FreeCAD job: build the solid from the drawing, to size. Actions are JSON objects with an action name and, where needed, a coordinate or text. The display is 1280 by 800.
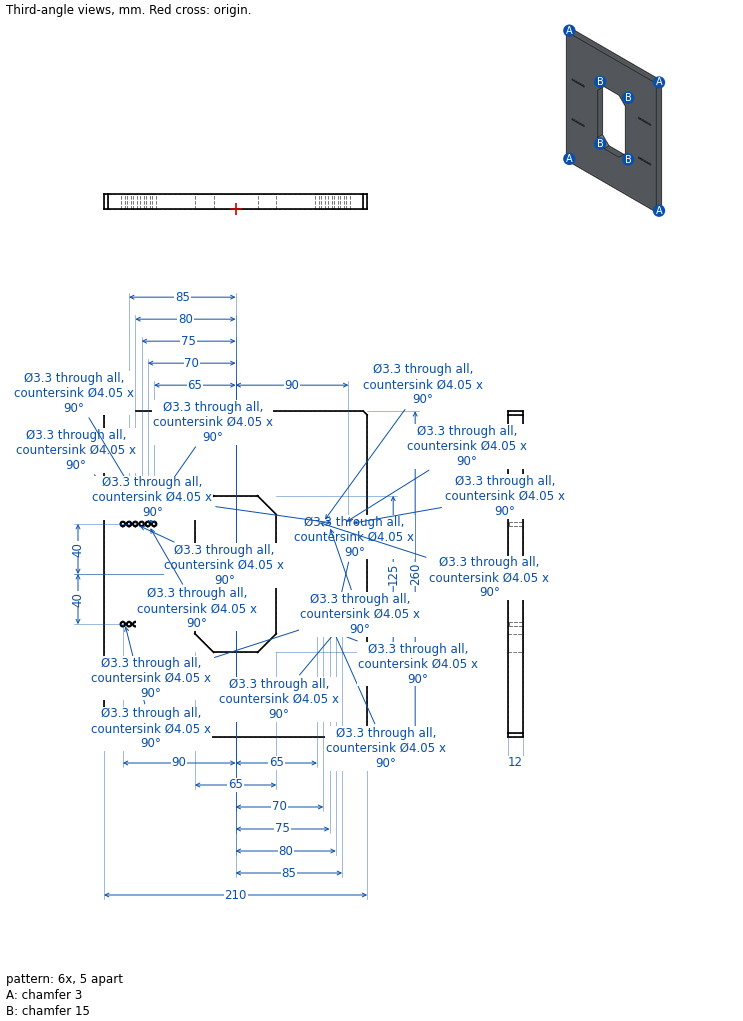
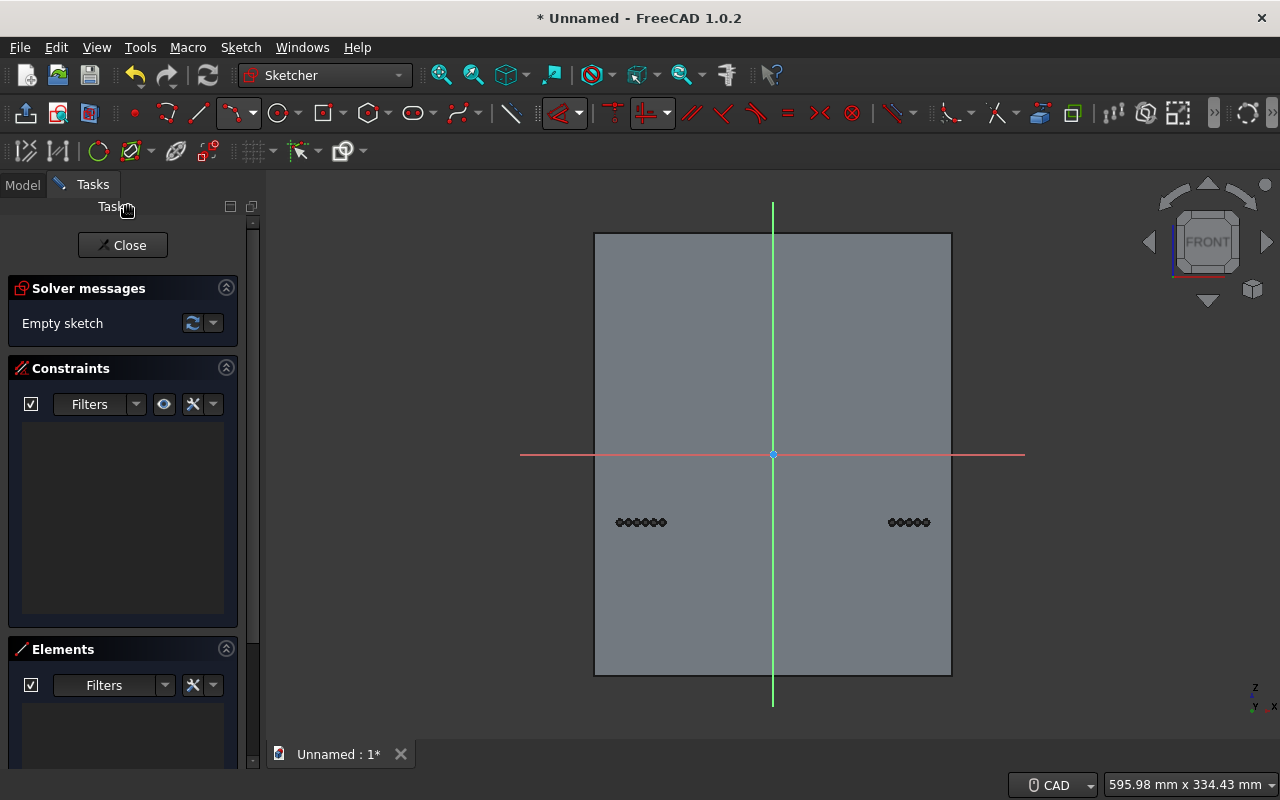
{"action": "scroll", "coordinate": [893, 526], "scroll_direction": "up", "scroll_amount": 15}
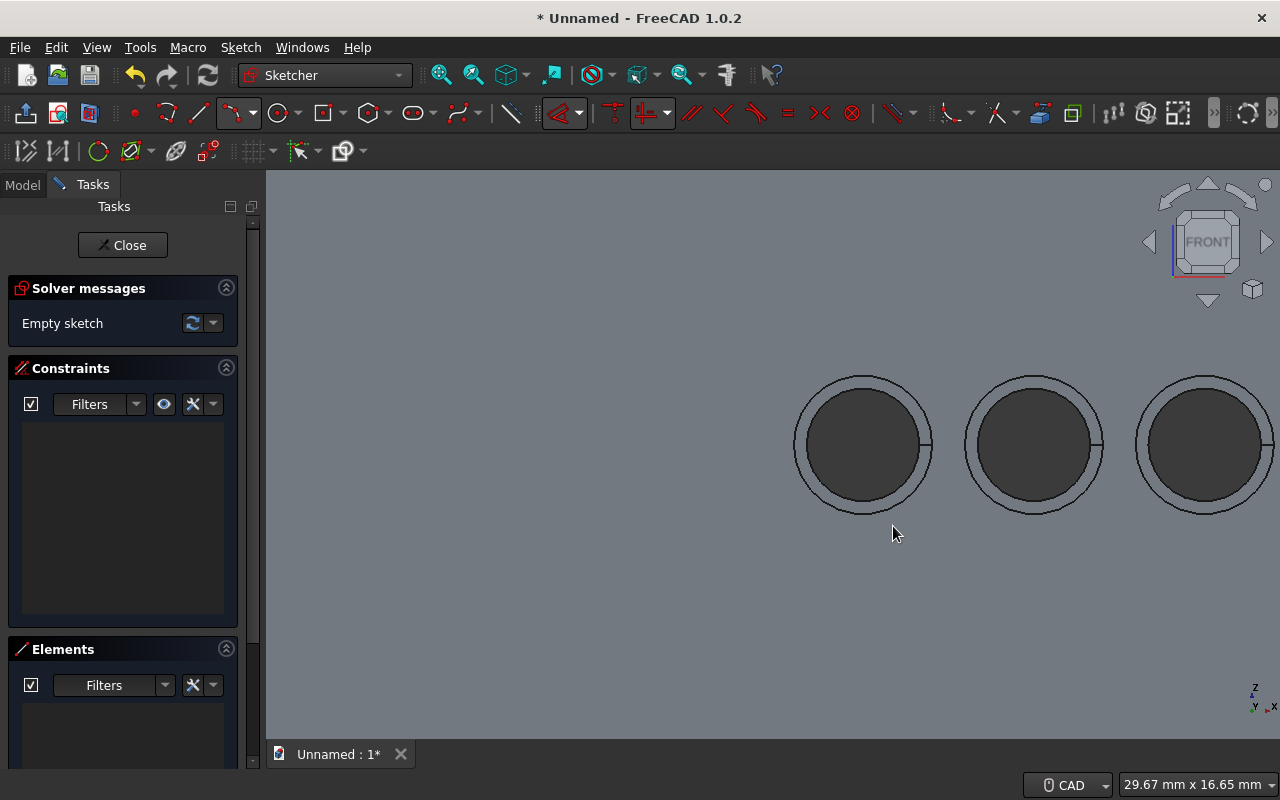
{"action": "scroll", "coordinate": [687, 441], "scroll_direction": "up", "scroll_amount": 6}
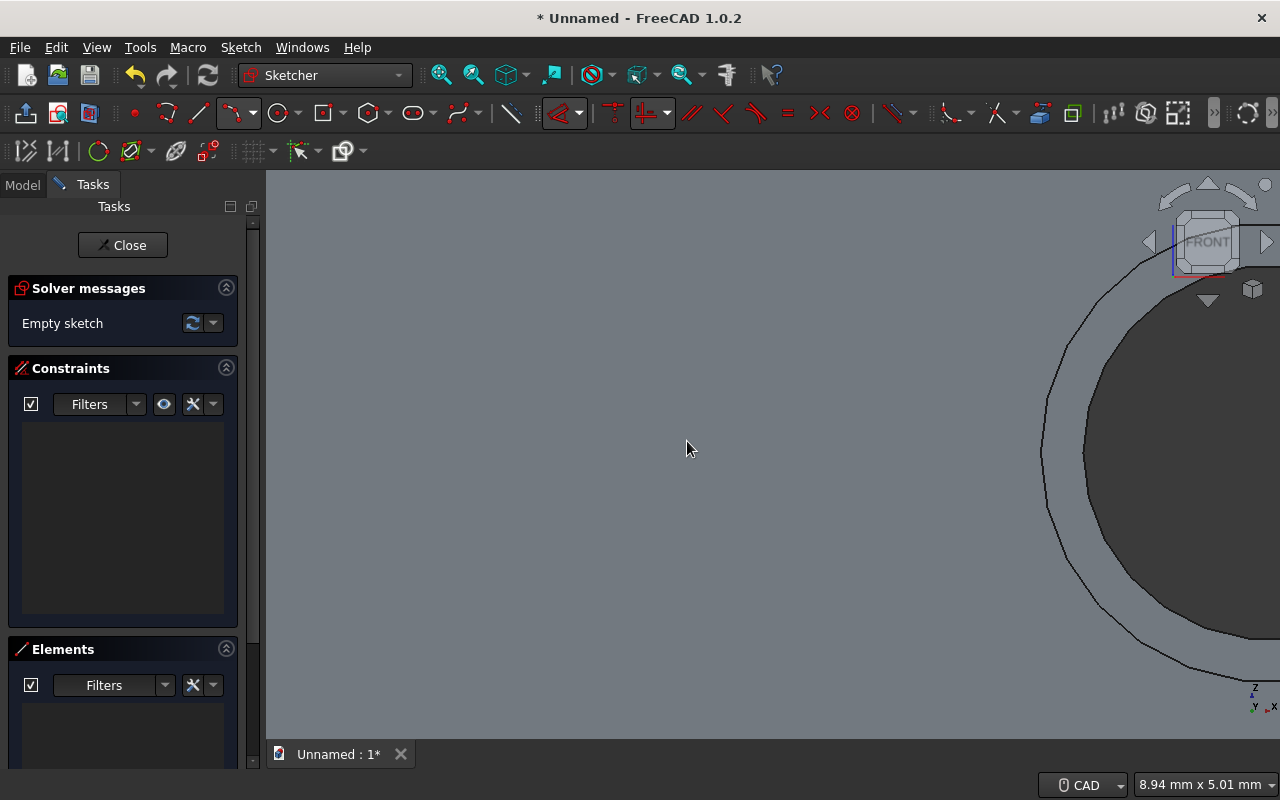
{"action": "left_click", "coordinate": [278, 114]}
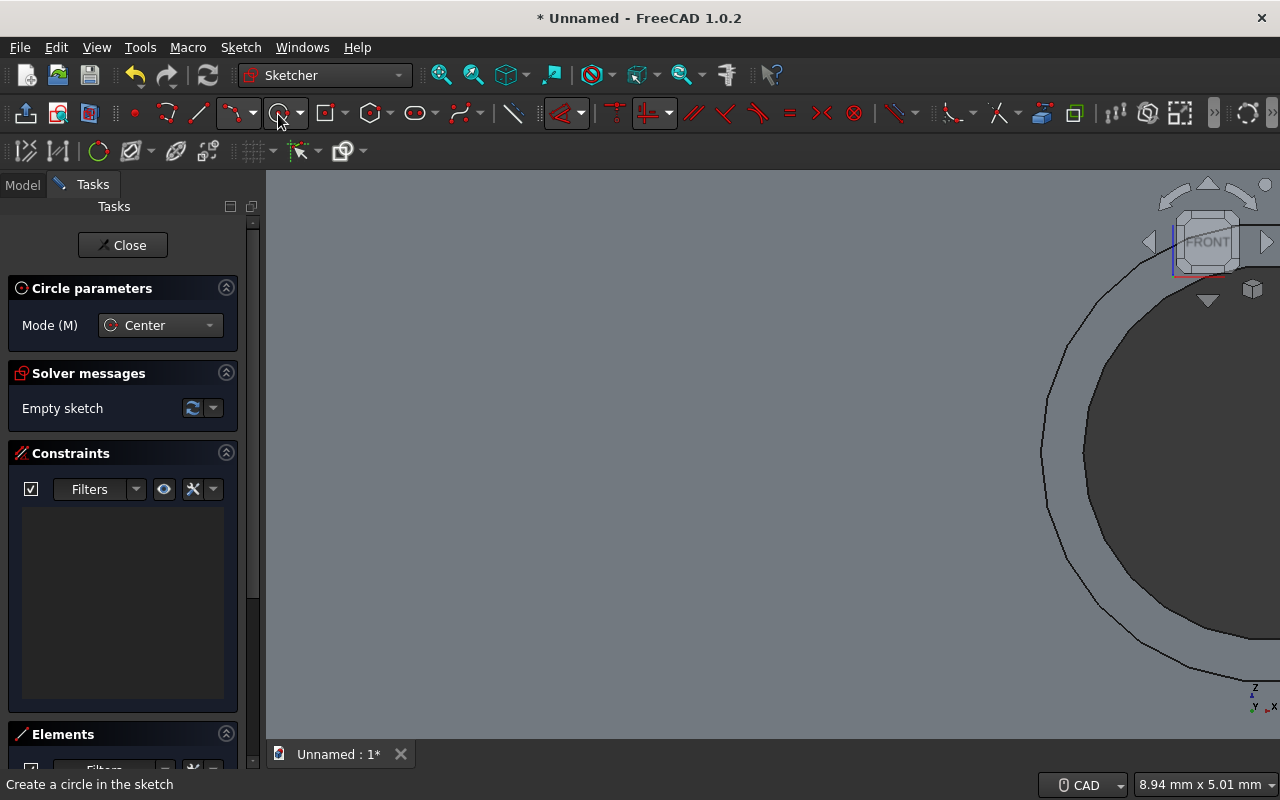
{"action": "left_click", "coordinate": [703, 453]}
{"action": "mouse_move", "coordinate": [836, 320]}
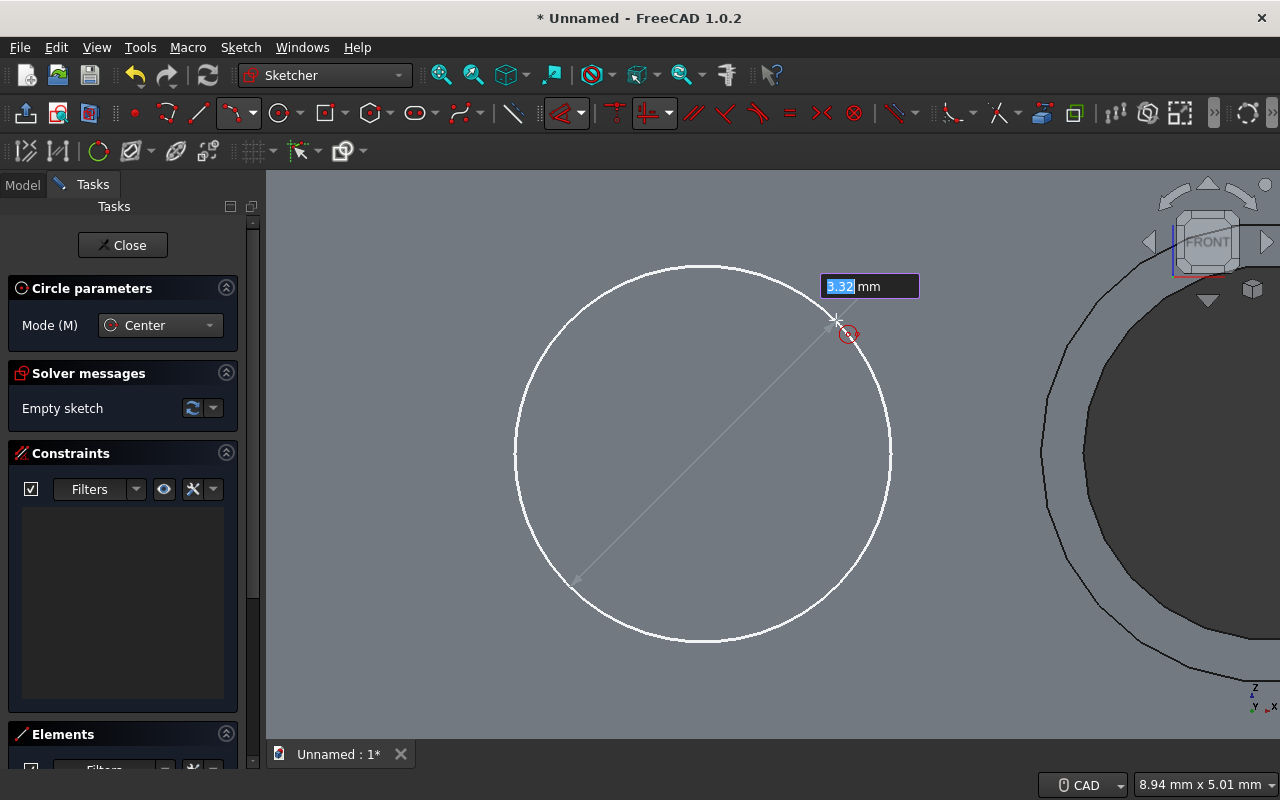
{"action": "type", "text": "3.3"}
{"action": "key", "text": "Return"}
{"action": "key", "text": "Escape"}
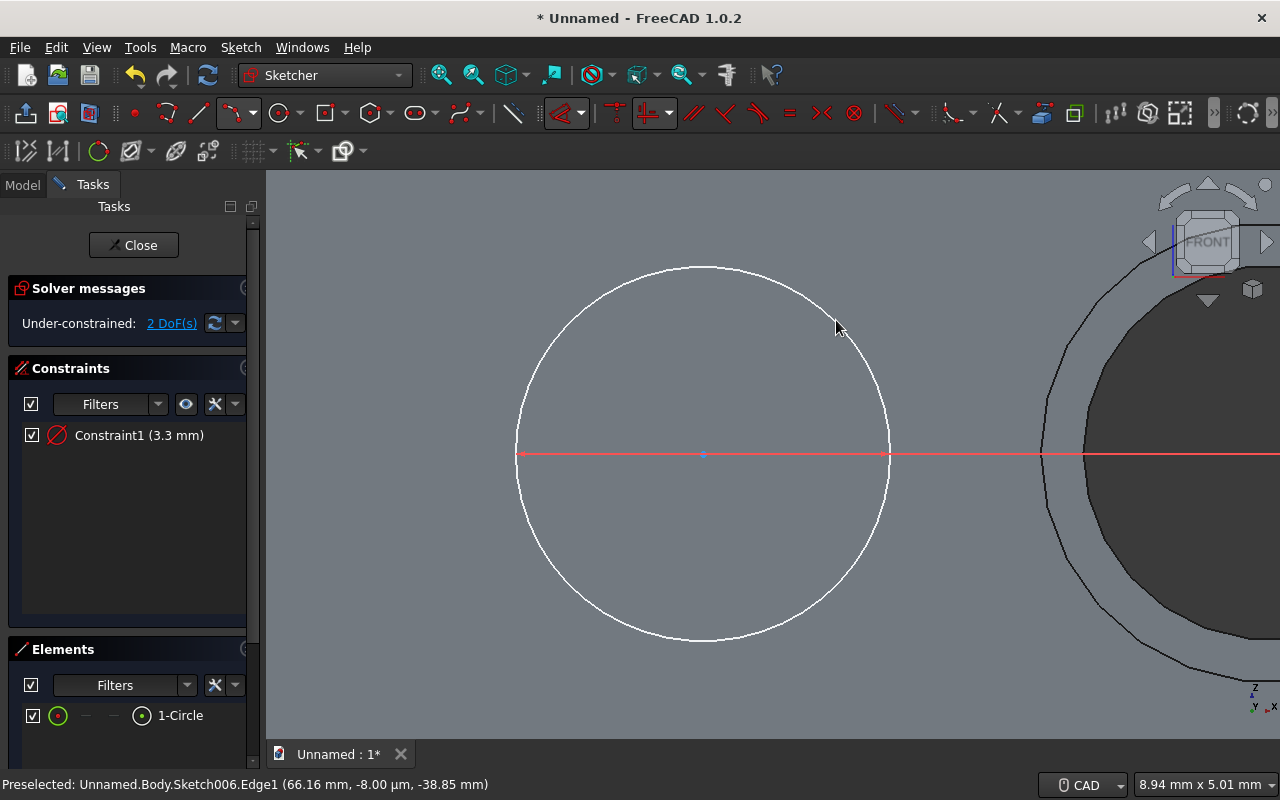
{"action": "left_click", "coordinate": [703, 454]}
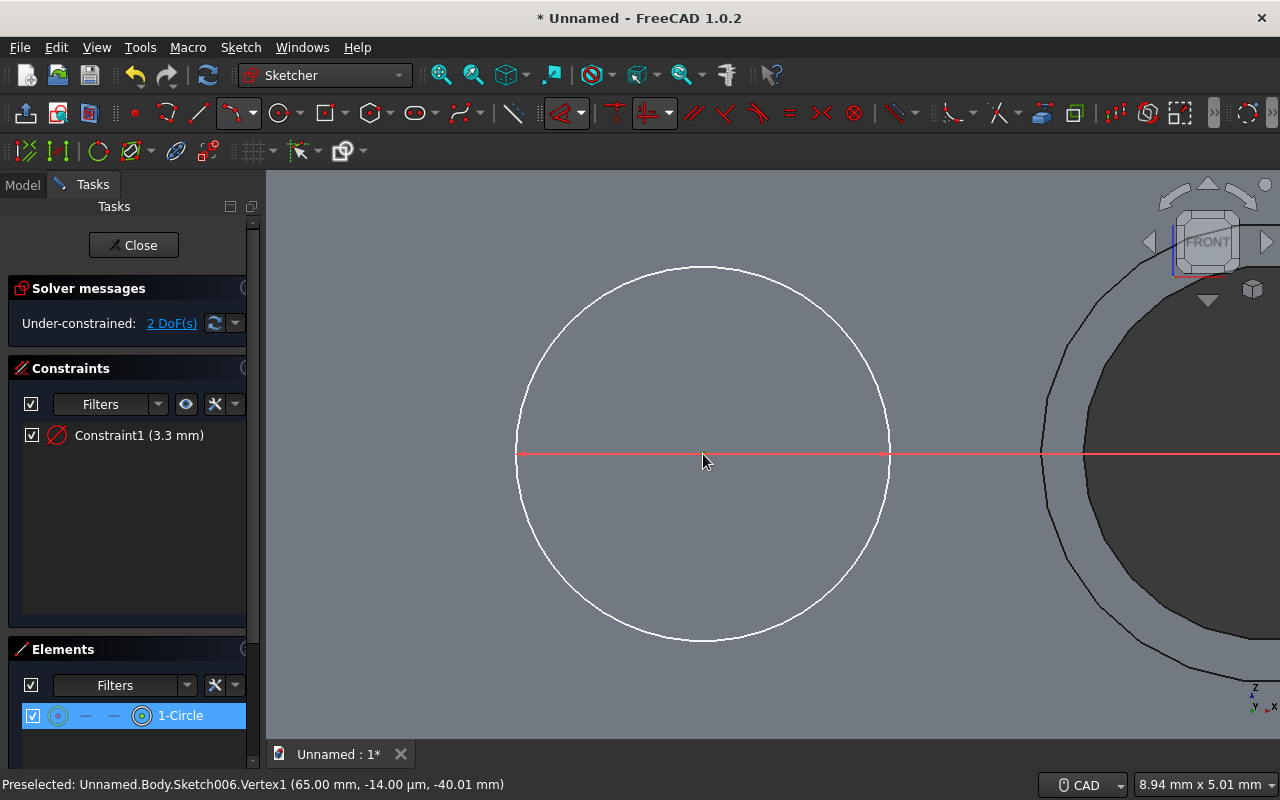
{"action": "left_click", "coordinate": [584, 114]}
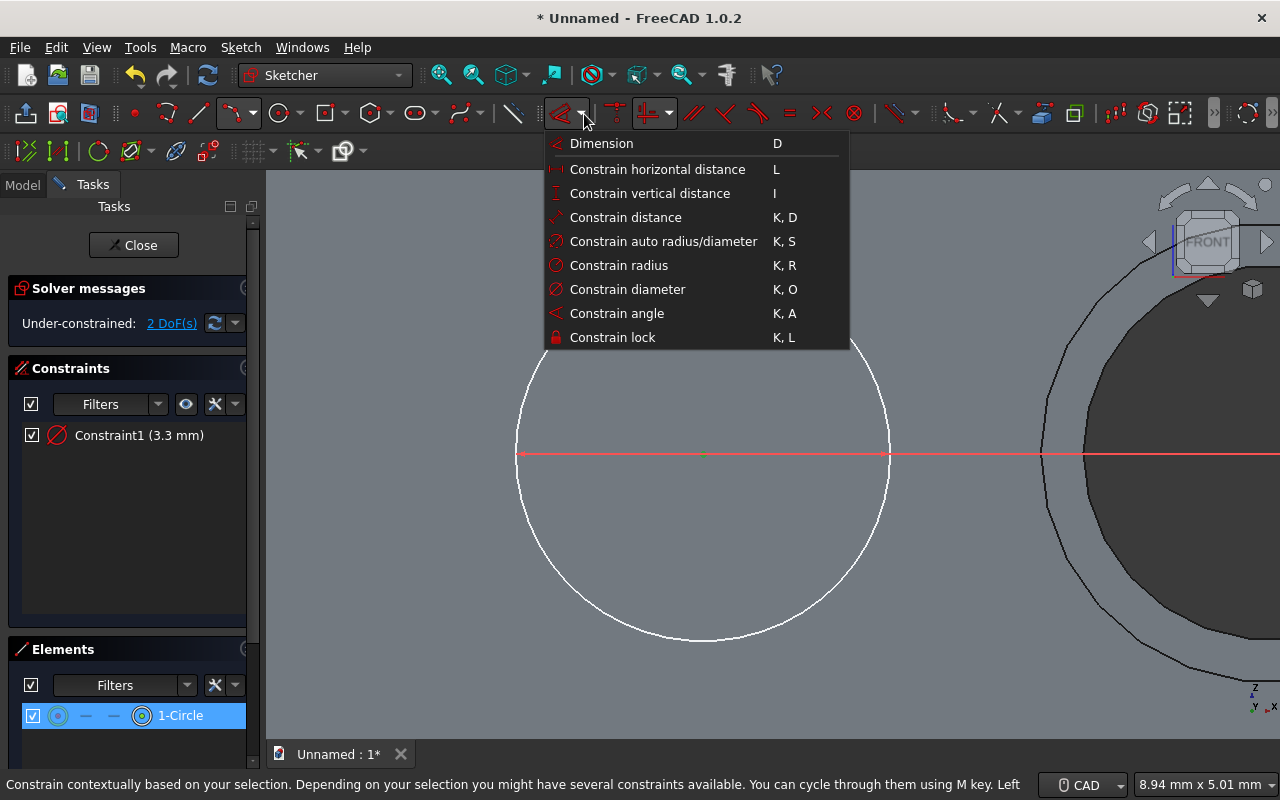
{"action": "left_click", "coordinate": [697, 169]}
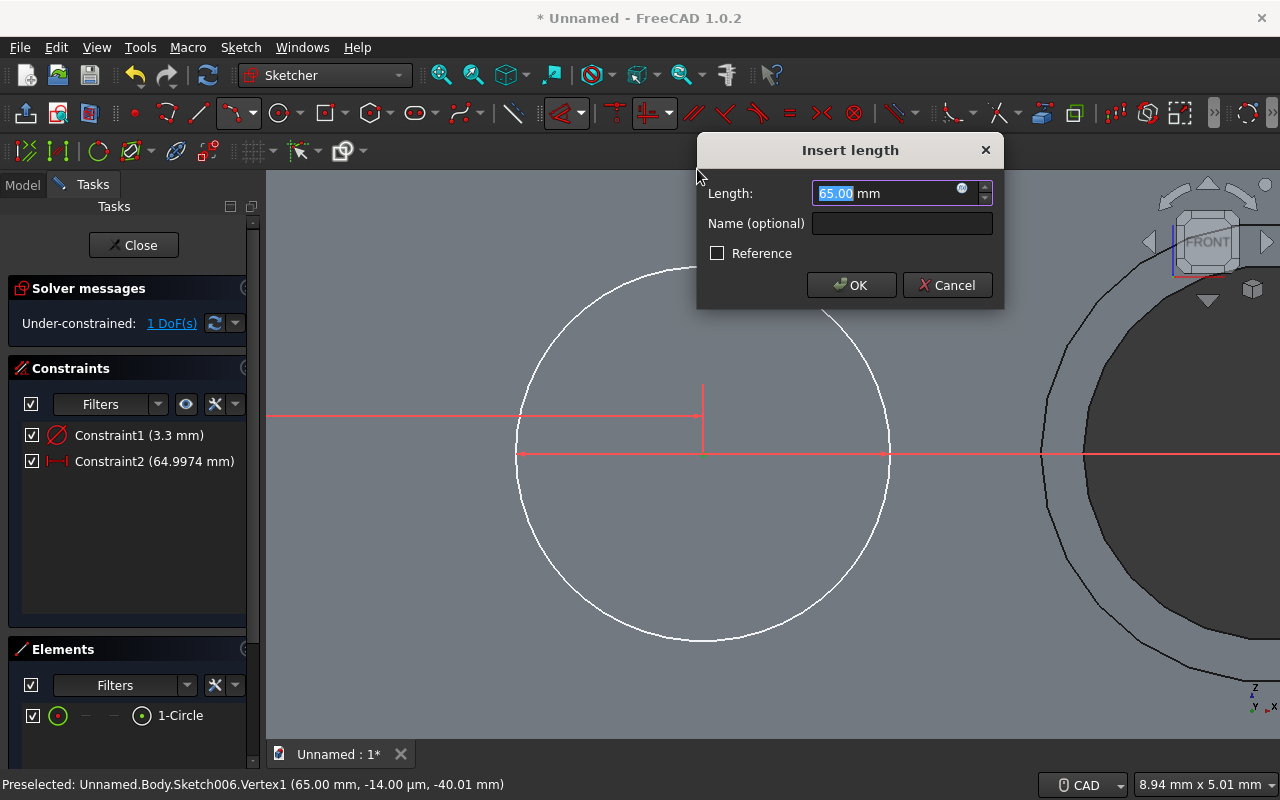
{"action": "type", "text": "65"}
{"action": "key", "text": "Return"}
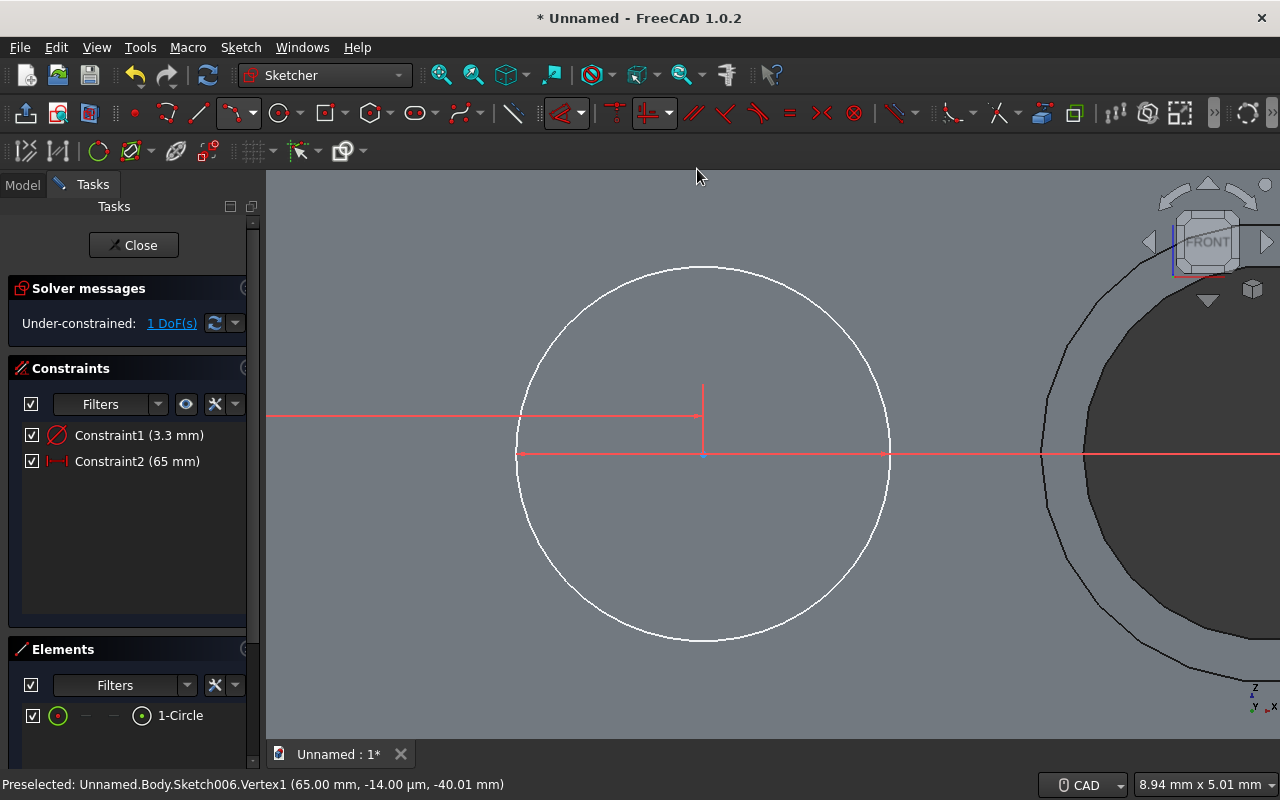
{"action": "left_click", "coordinate": [703, 454]}